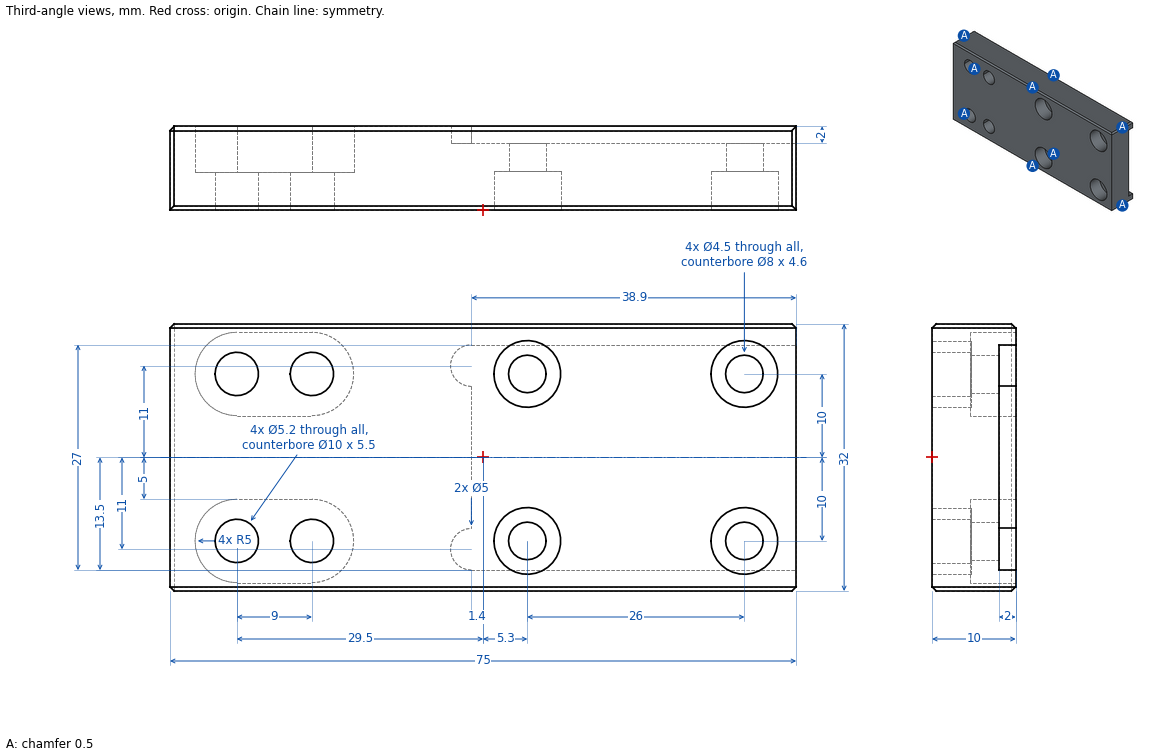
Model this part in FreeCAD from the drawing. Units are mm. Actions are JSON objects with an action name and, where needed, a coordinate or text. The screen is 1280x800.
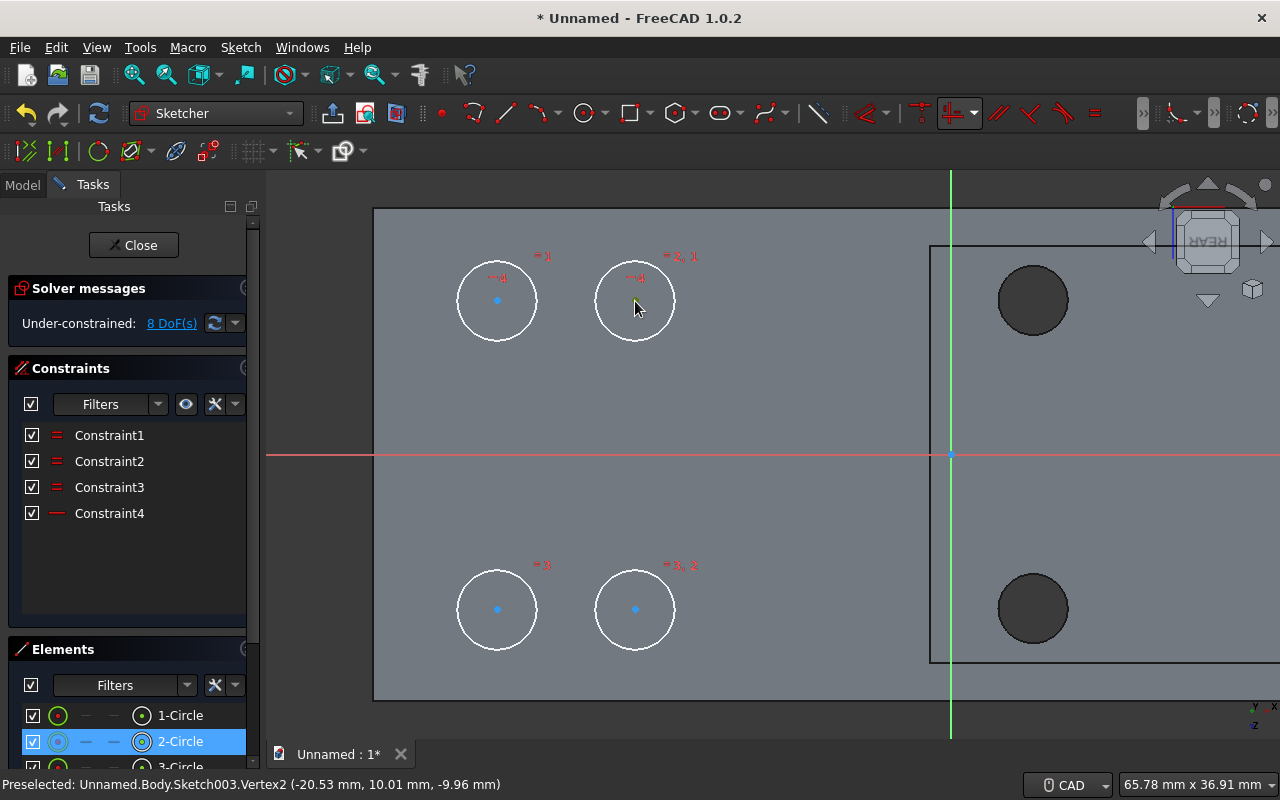
{"action": "left_click", "coordinate": [635, 610]}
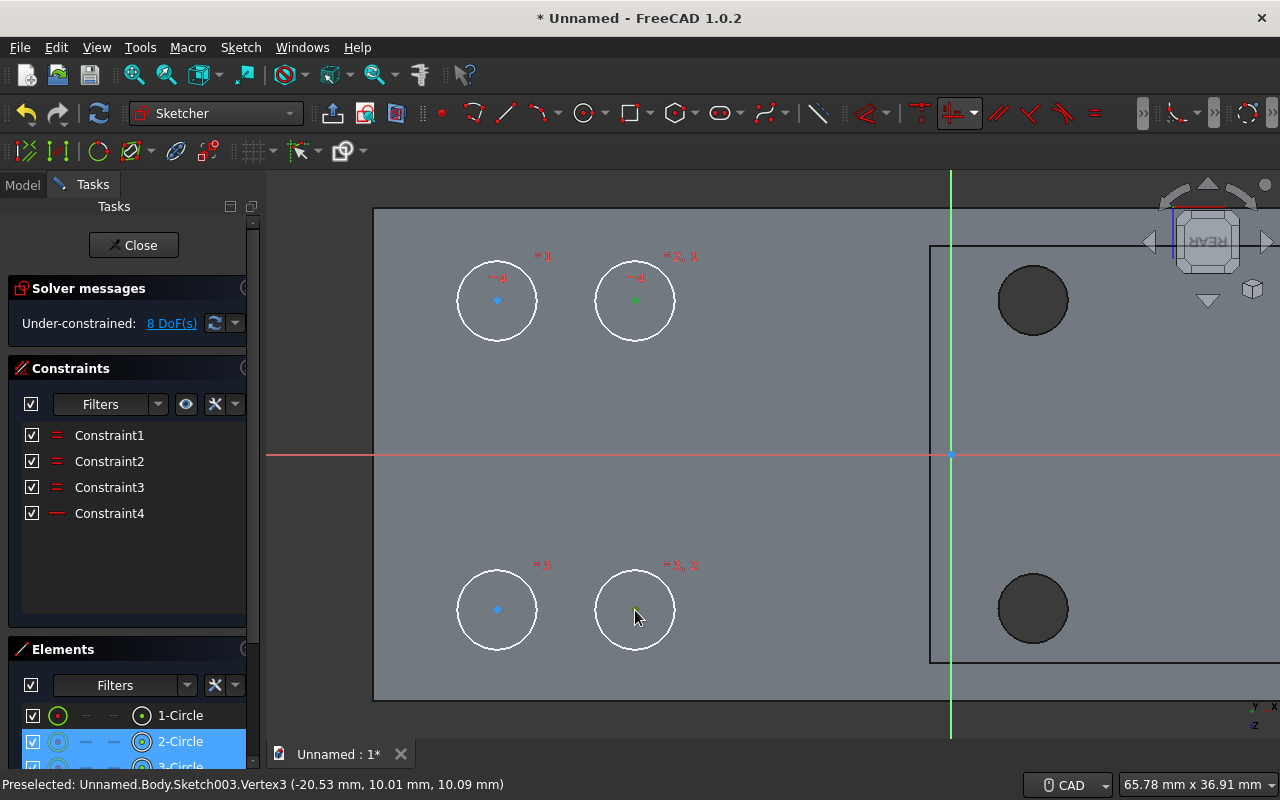
{"action": "left_click", "coordinate": [976, 114]}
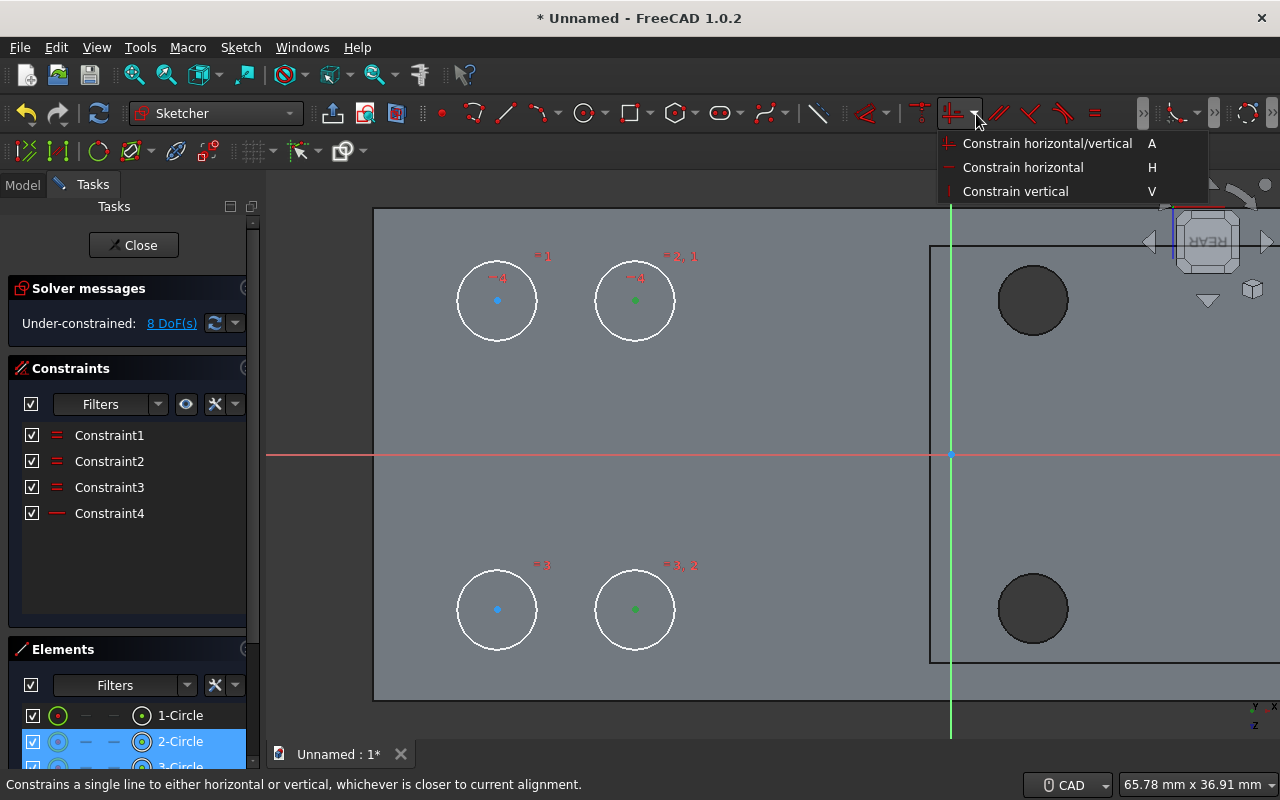
{"action": "left_click", "coordinate": [1073, 191]}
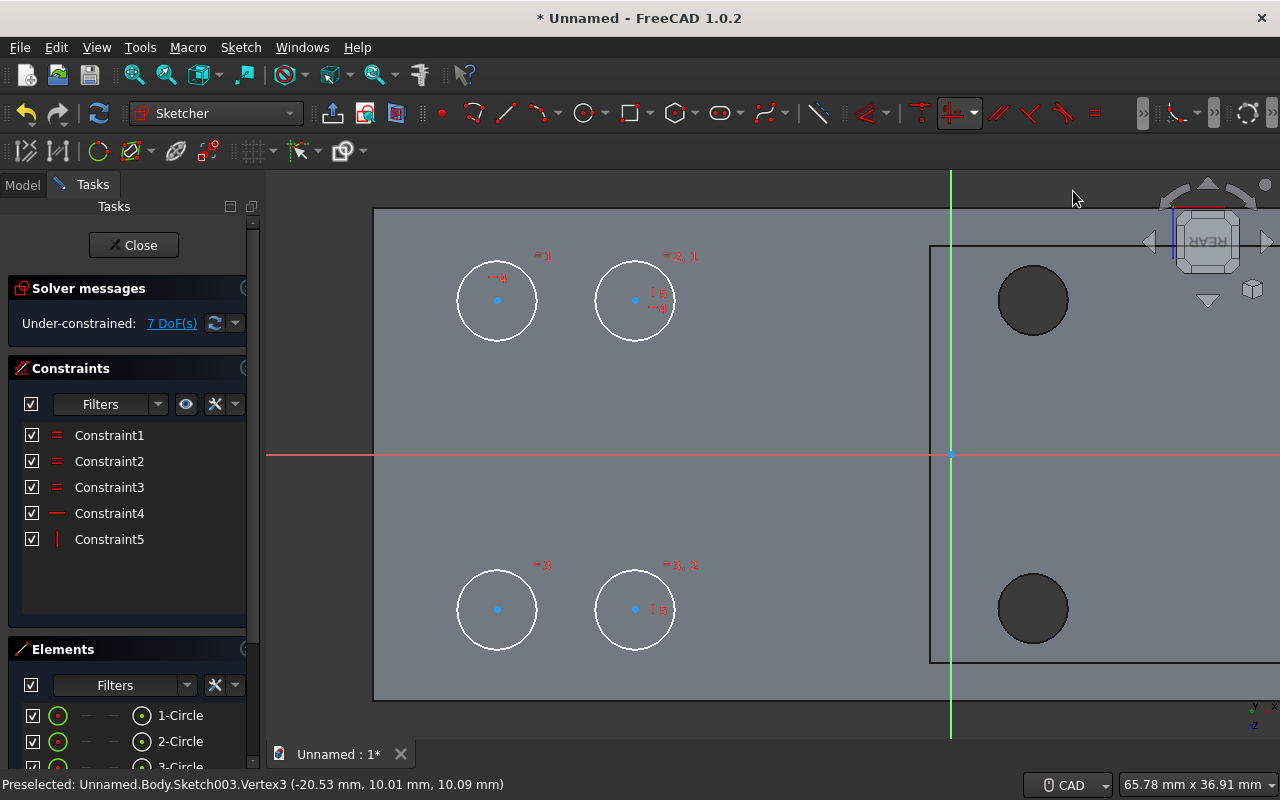
{"action": "left_click", "coordinate": [497, 301]}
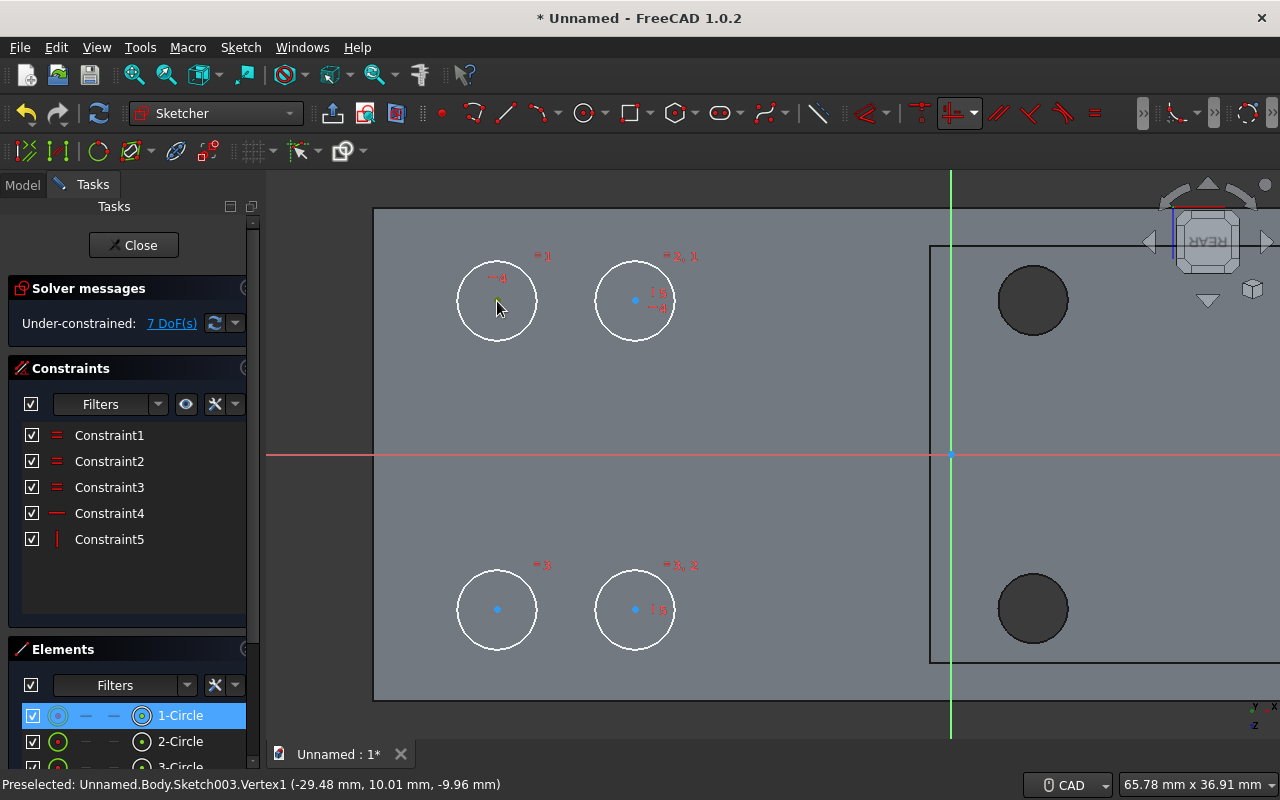
{"action": "left_click", "coordinate": [497, 610]}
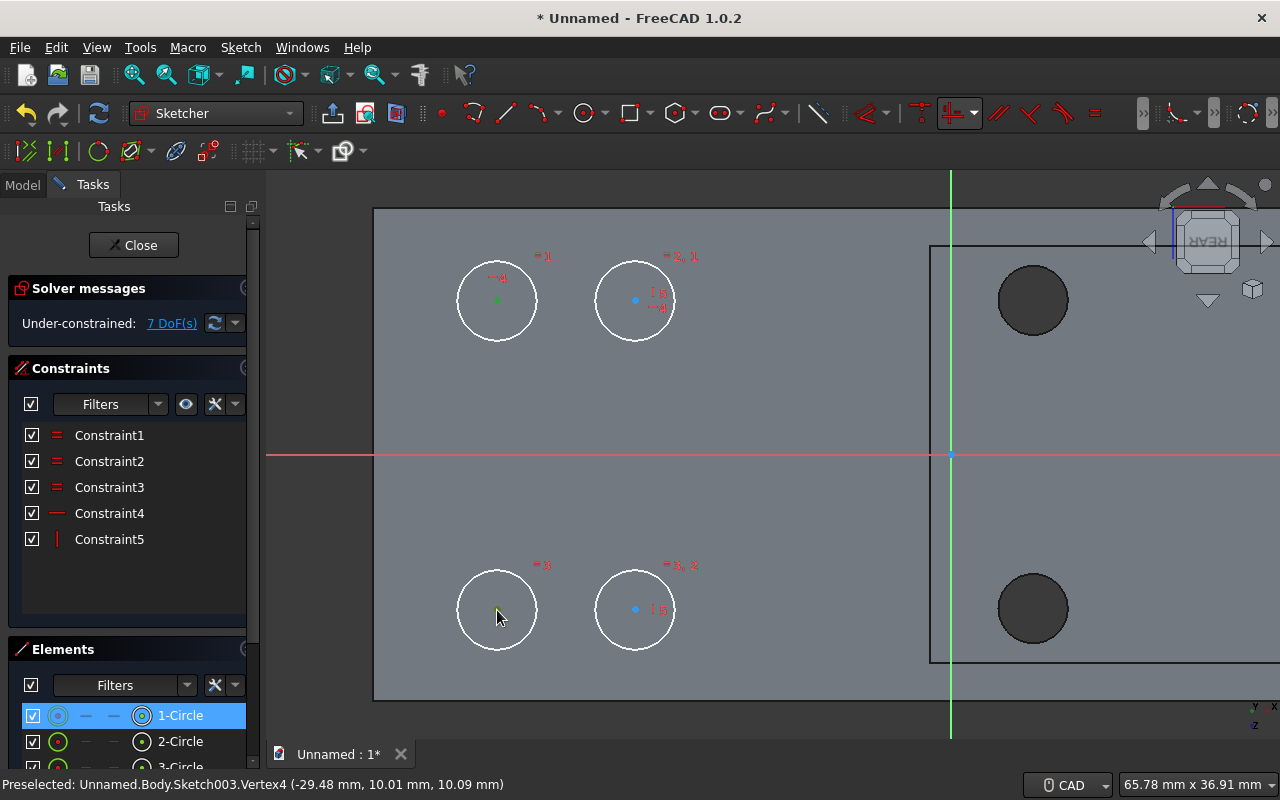
{"action": "left_click", "coordinate": [976, 114]}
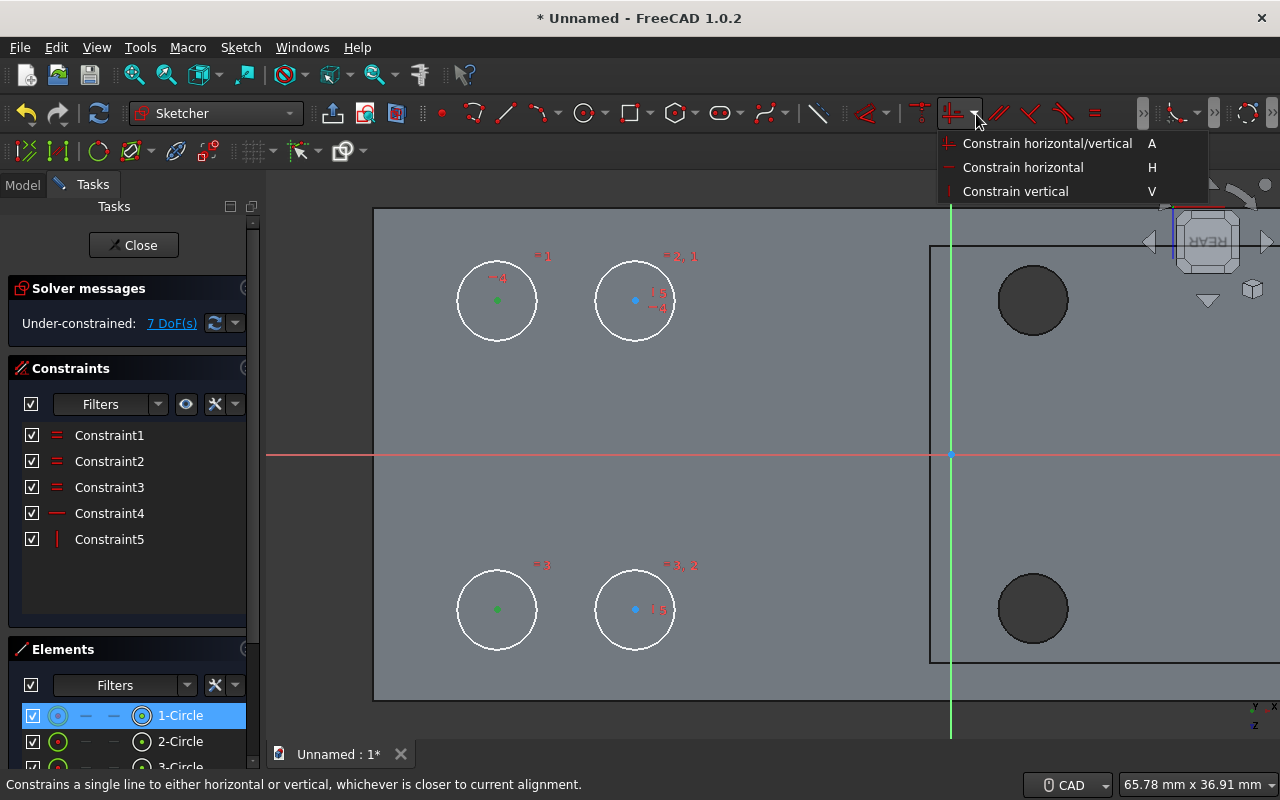
{"action": "left_click", "coordinate": [1073, 191]}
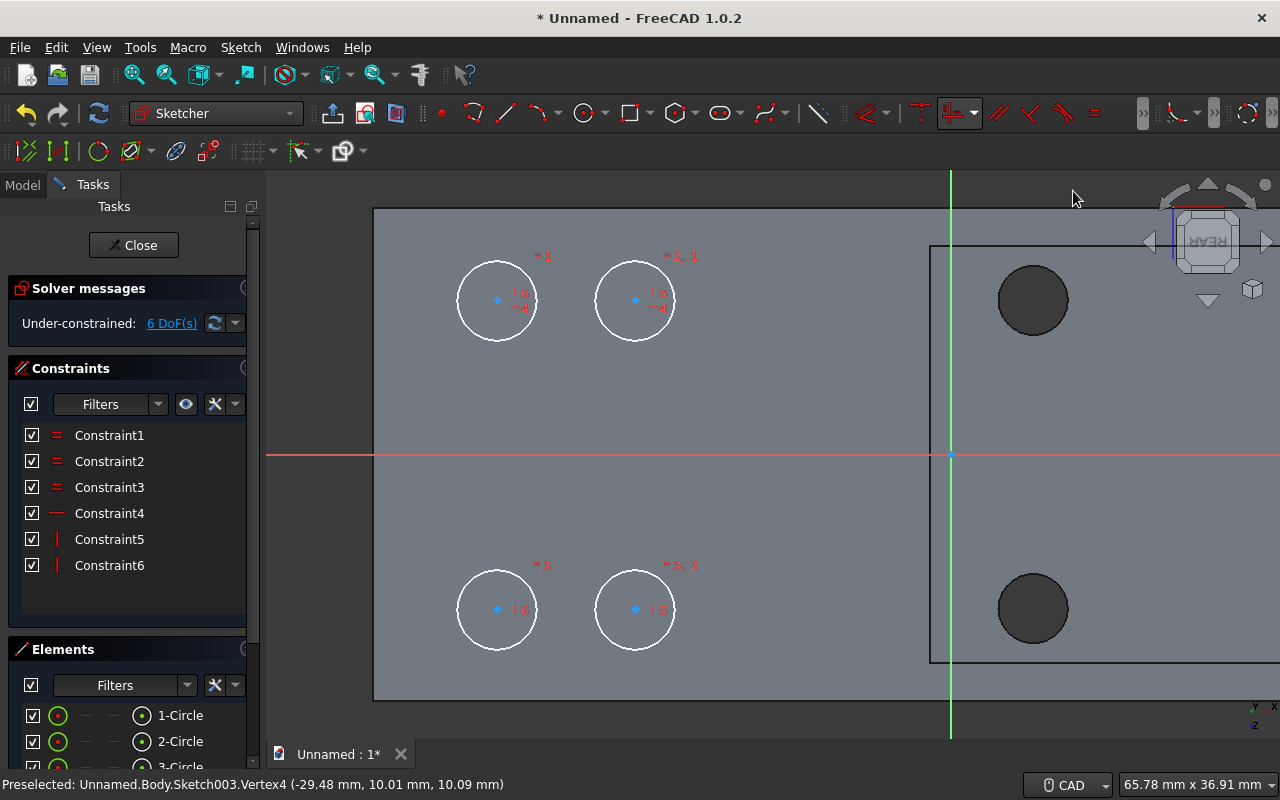
{"action": "left_click", "coordinate": [635, 610]}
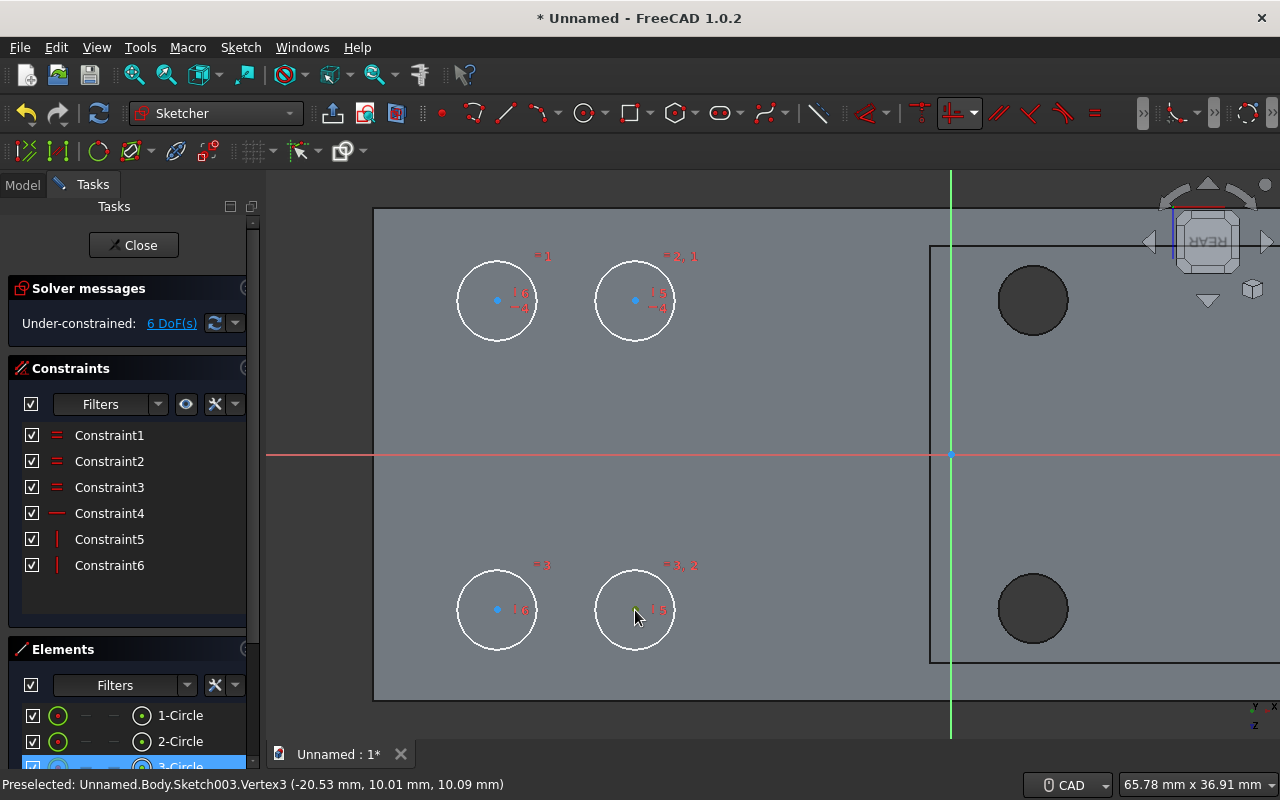
{"action": "left_click", "coordinate": [497, 610]}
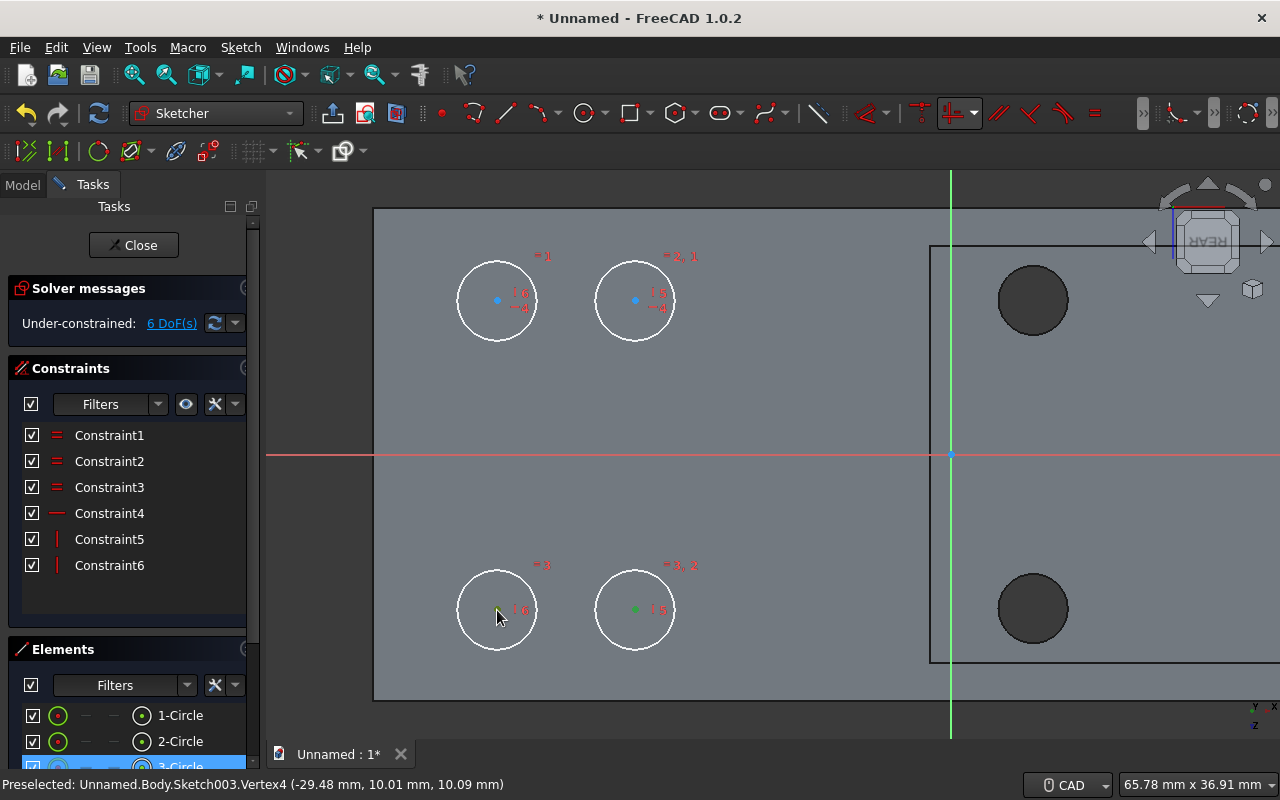
{"action": "left_click", "coordinate": [976, 114]}